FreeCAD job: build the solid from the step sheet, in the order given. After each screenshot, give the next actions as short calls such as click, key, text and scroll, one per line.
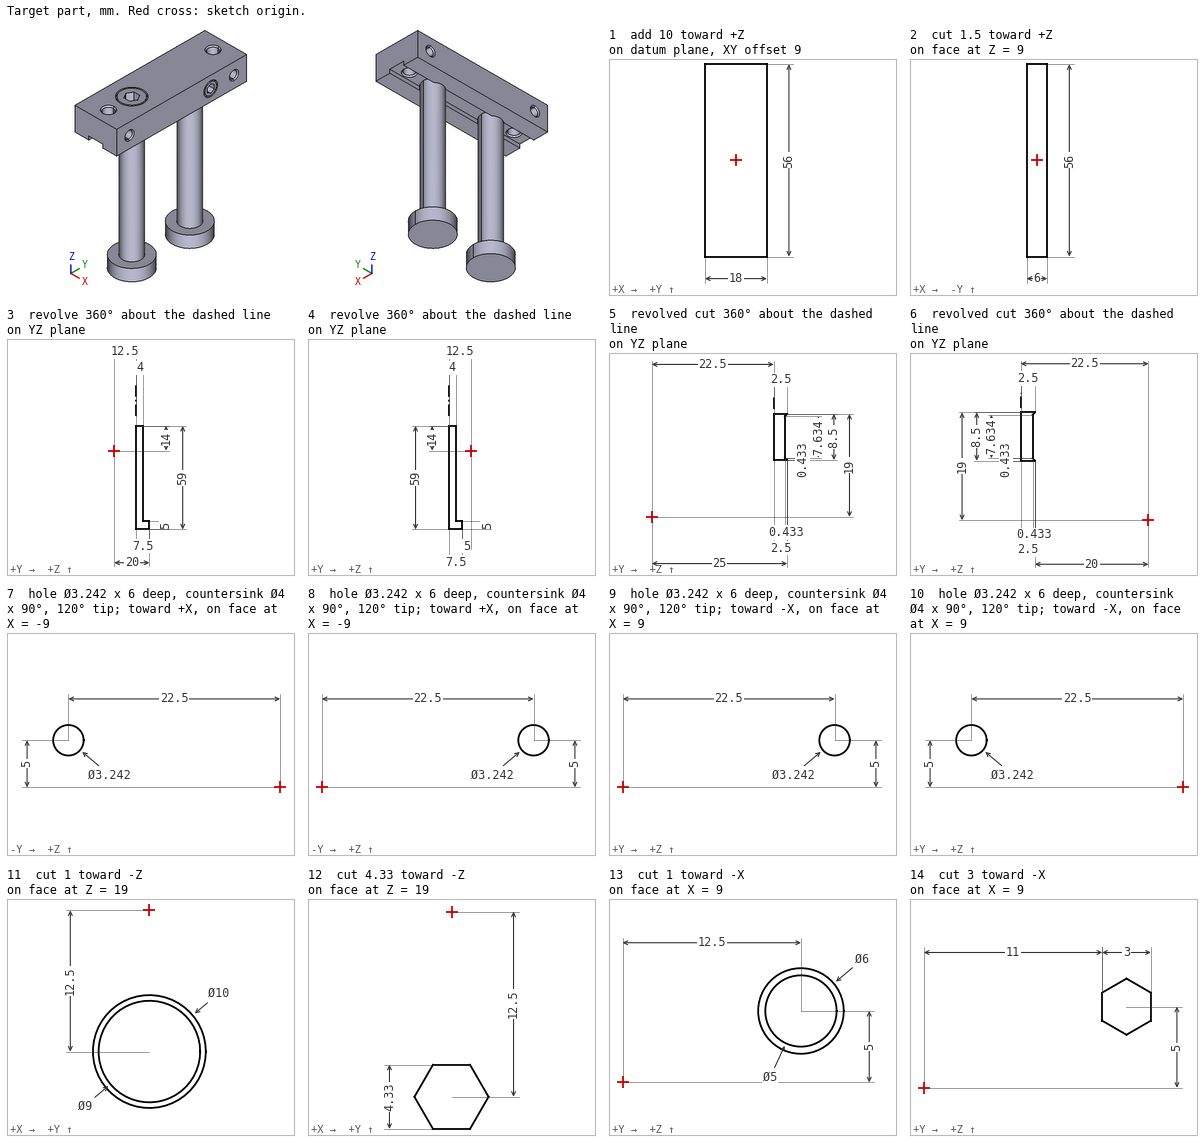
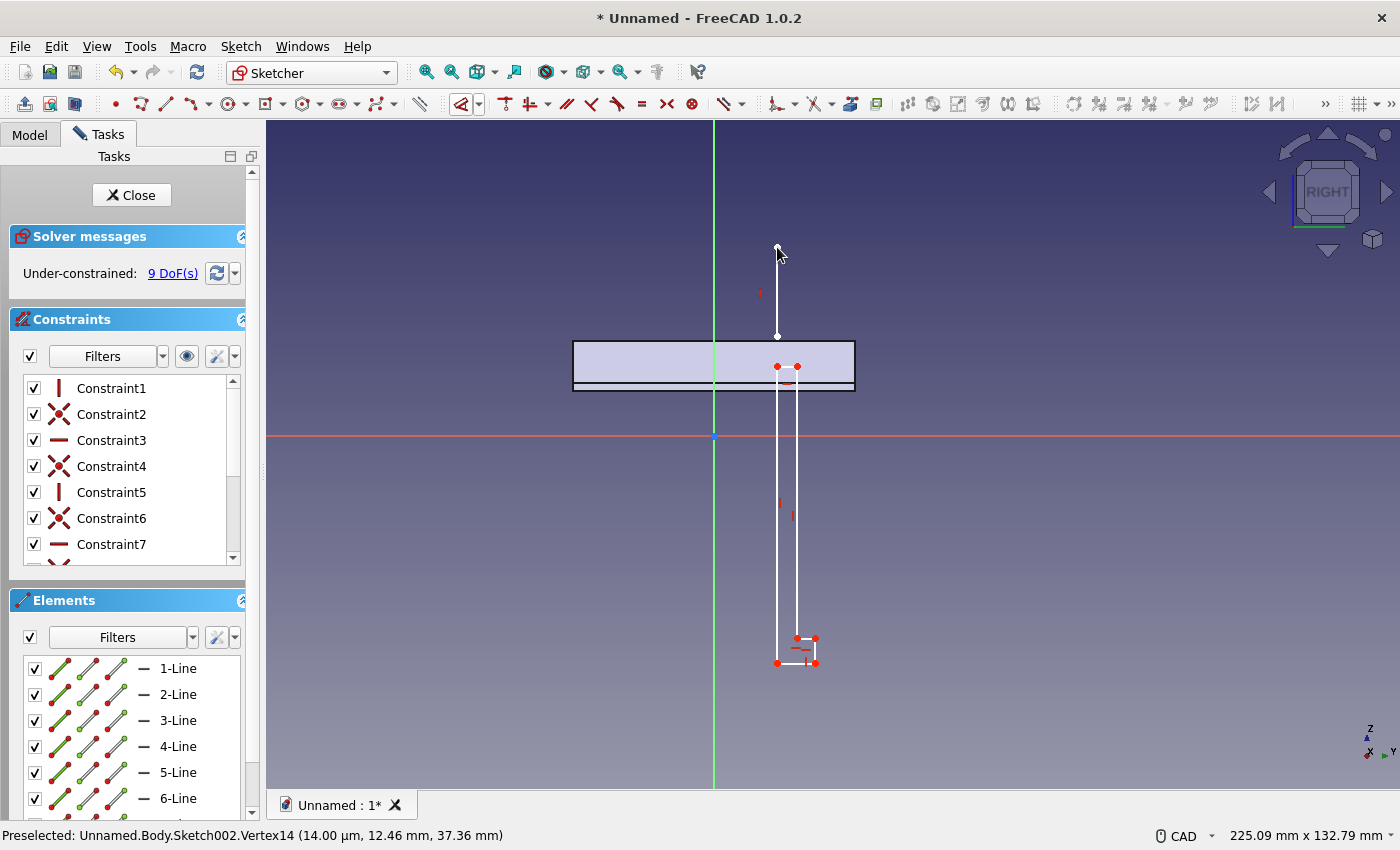
click(777, 310)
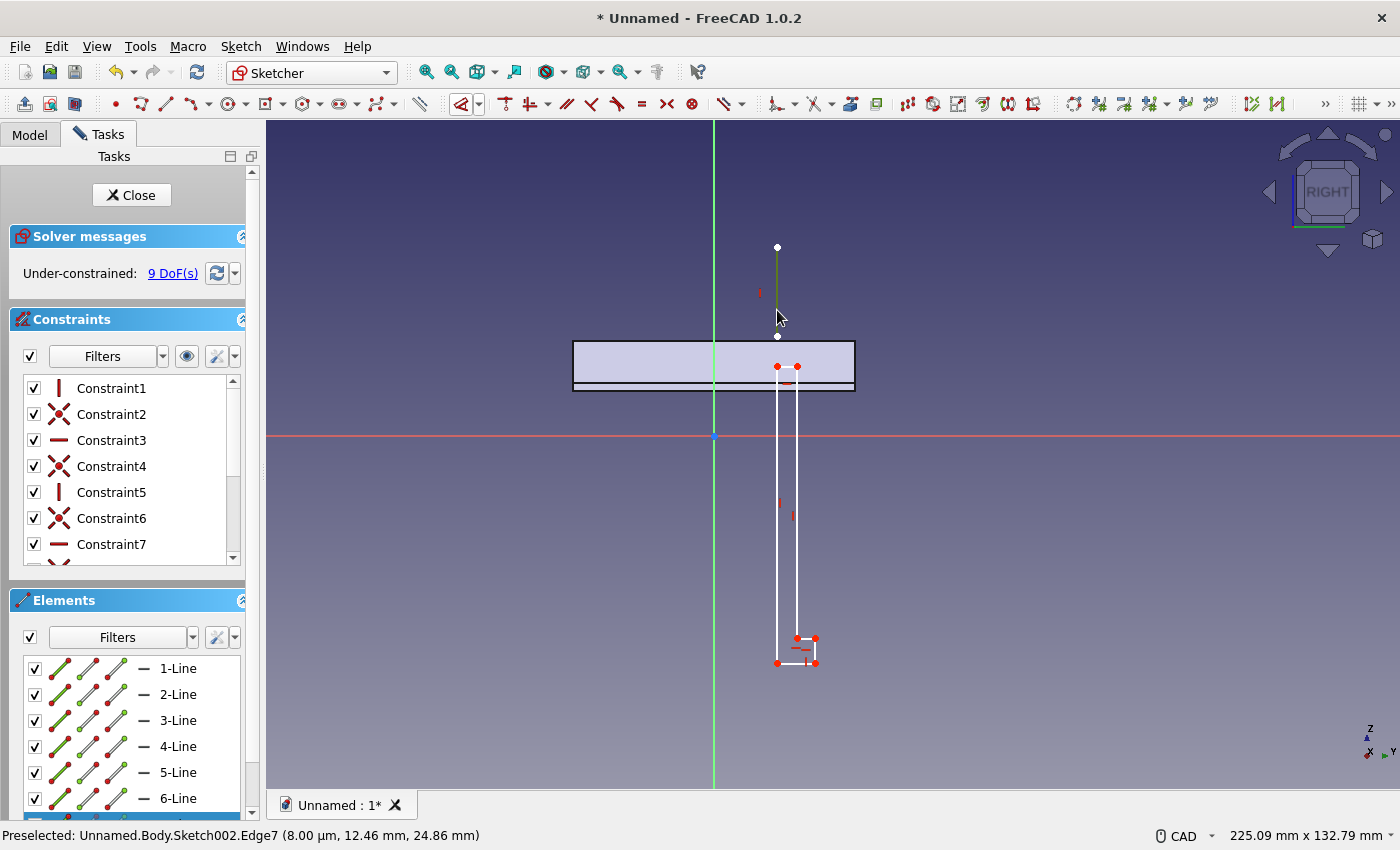
click(420, 104)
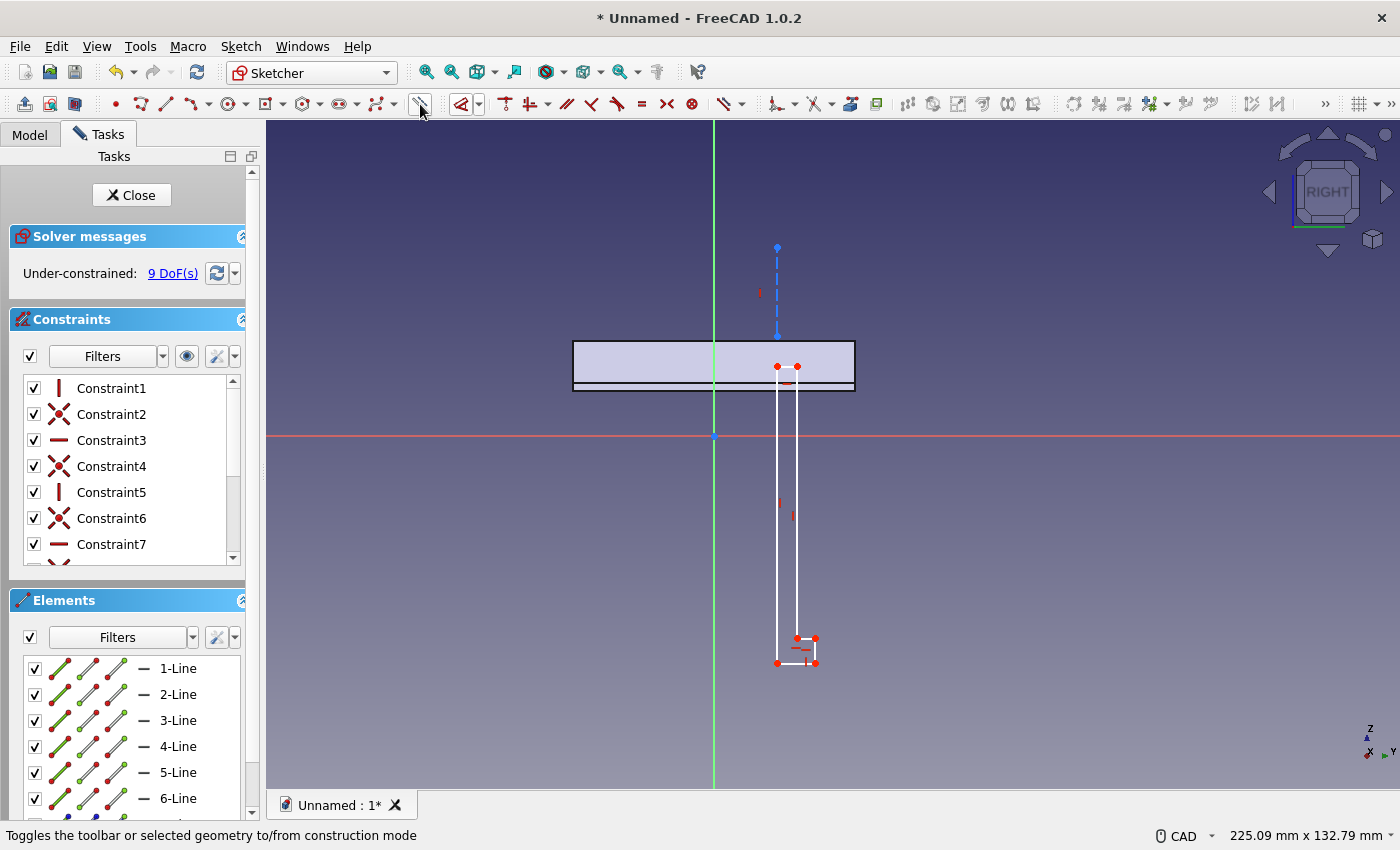
click(460, 104)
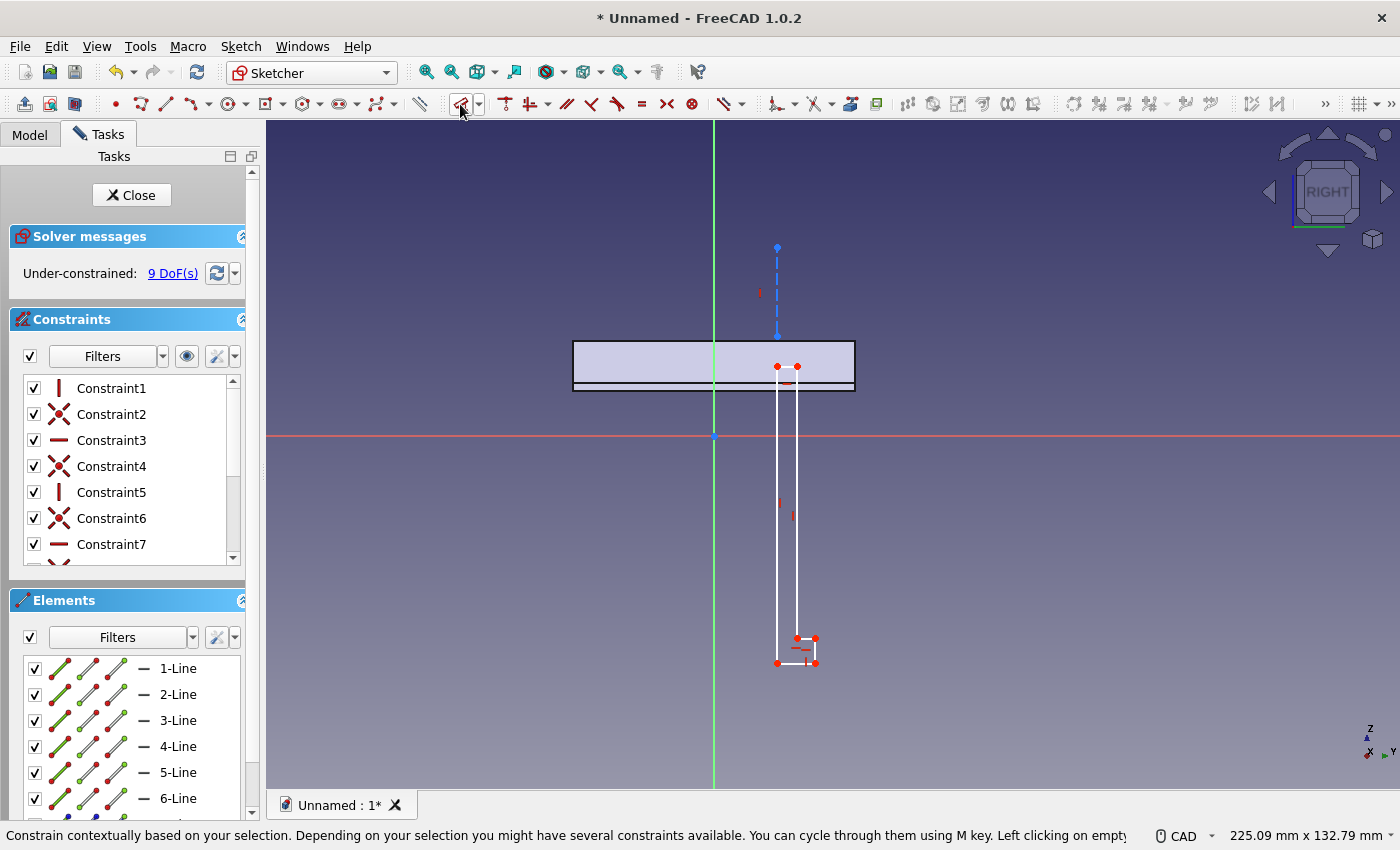
scroll(815, 654, up, 3)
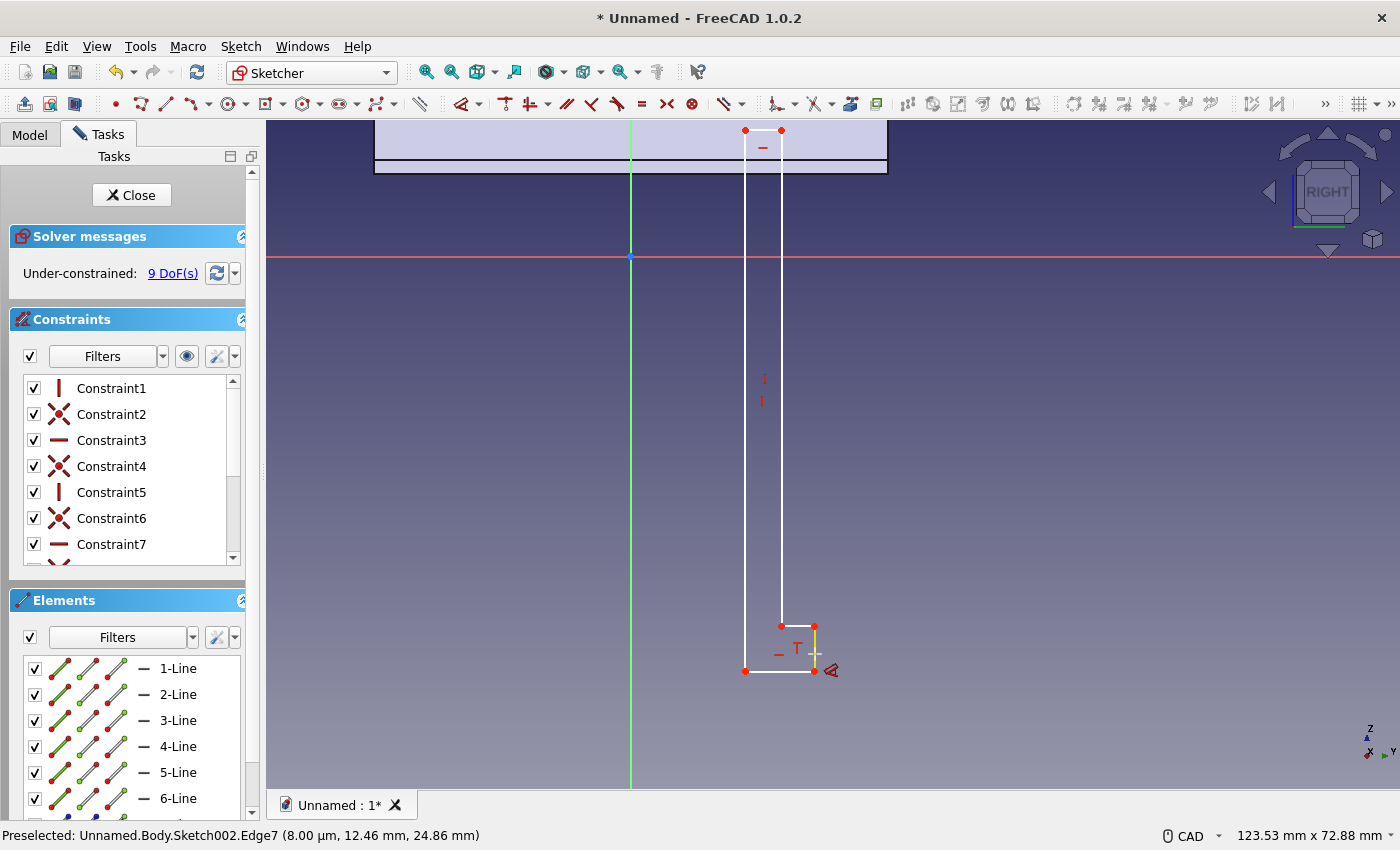
click(815, 653)
click(849, 649)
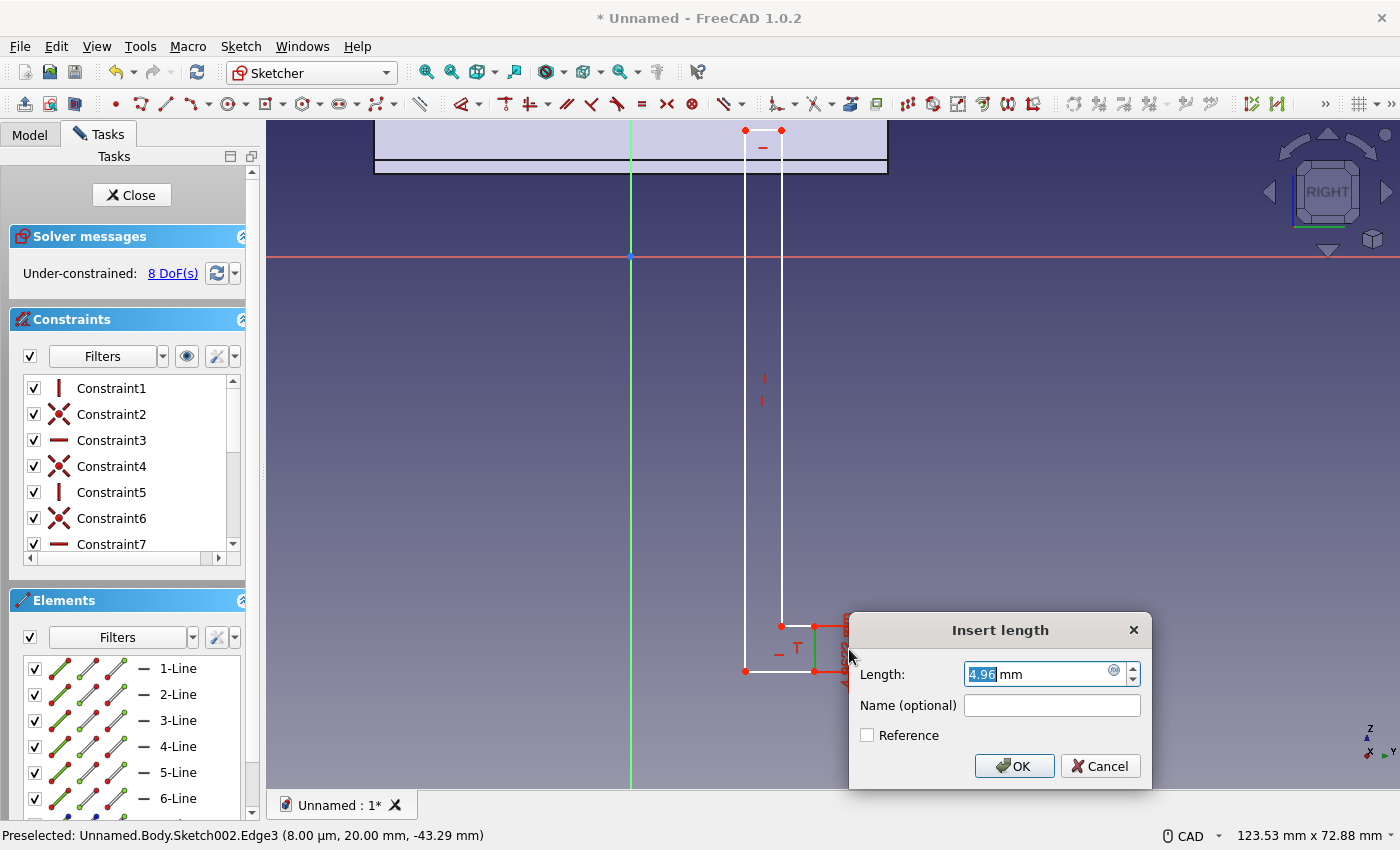
text(5)
key(Return)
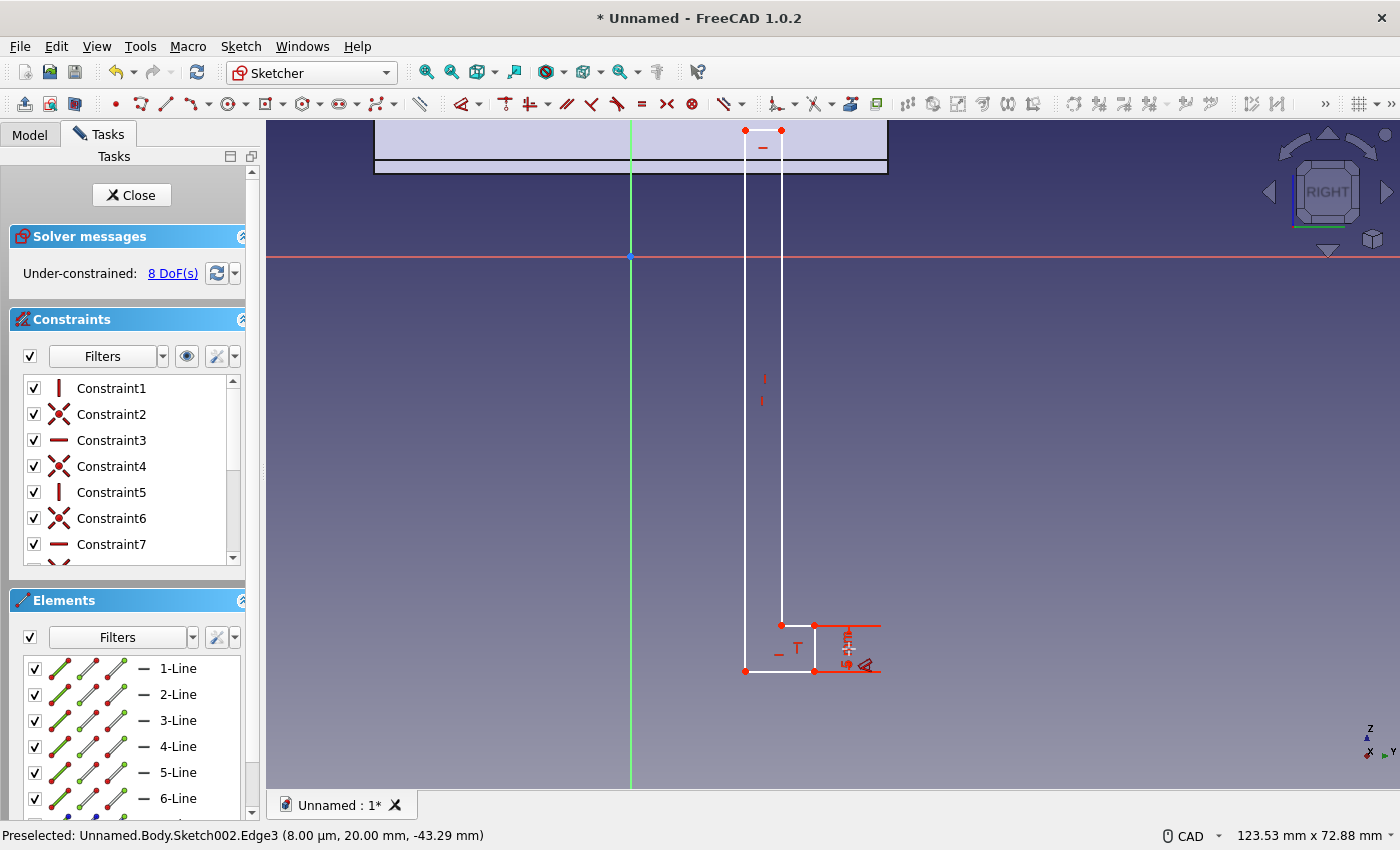
scroll(815, 654, down, 3)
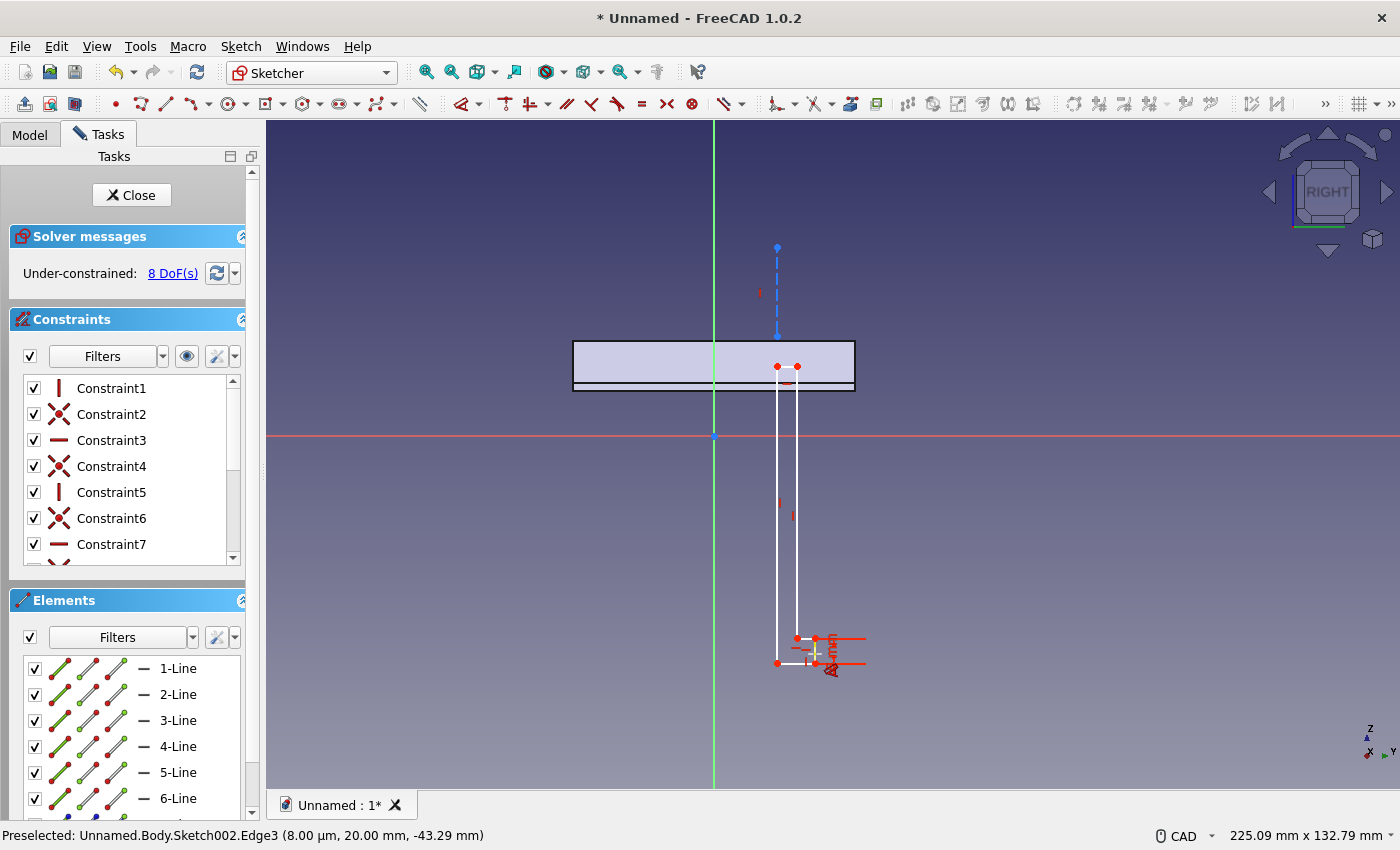
scroll(791, 367, up, 5)